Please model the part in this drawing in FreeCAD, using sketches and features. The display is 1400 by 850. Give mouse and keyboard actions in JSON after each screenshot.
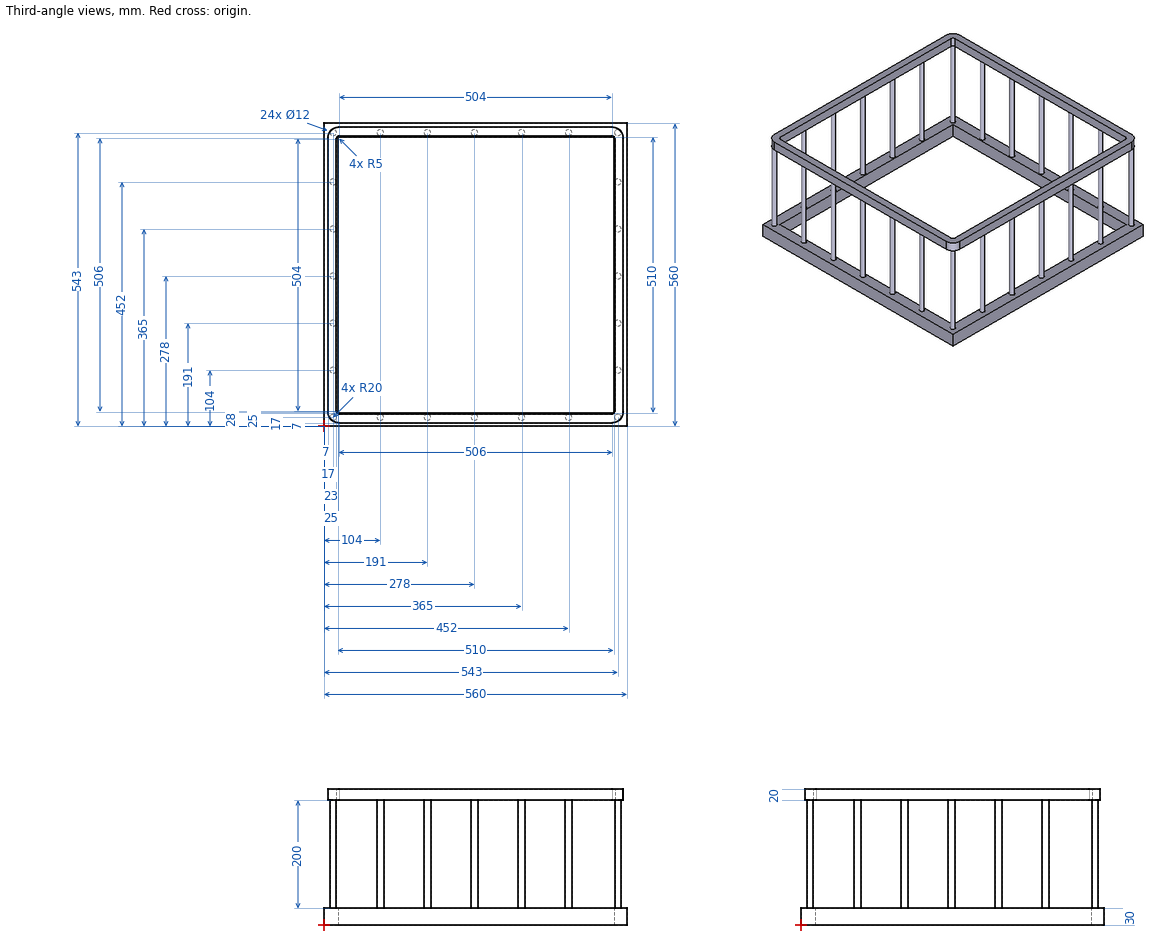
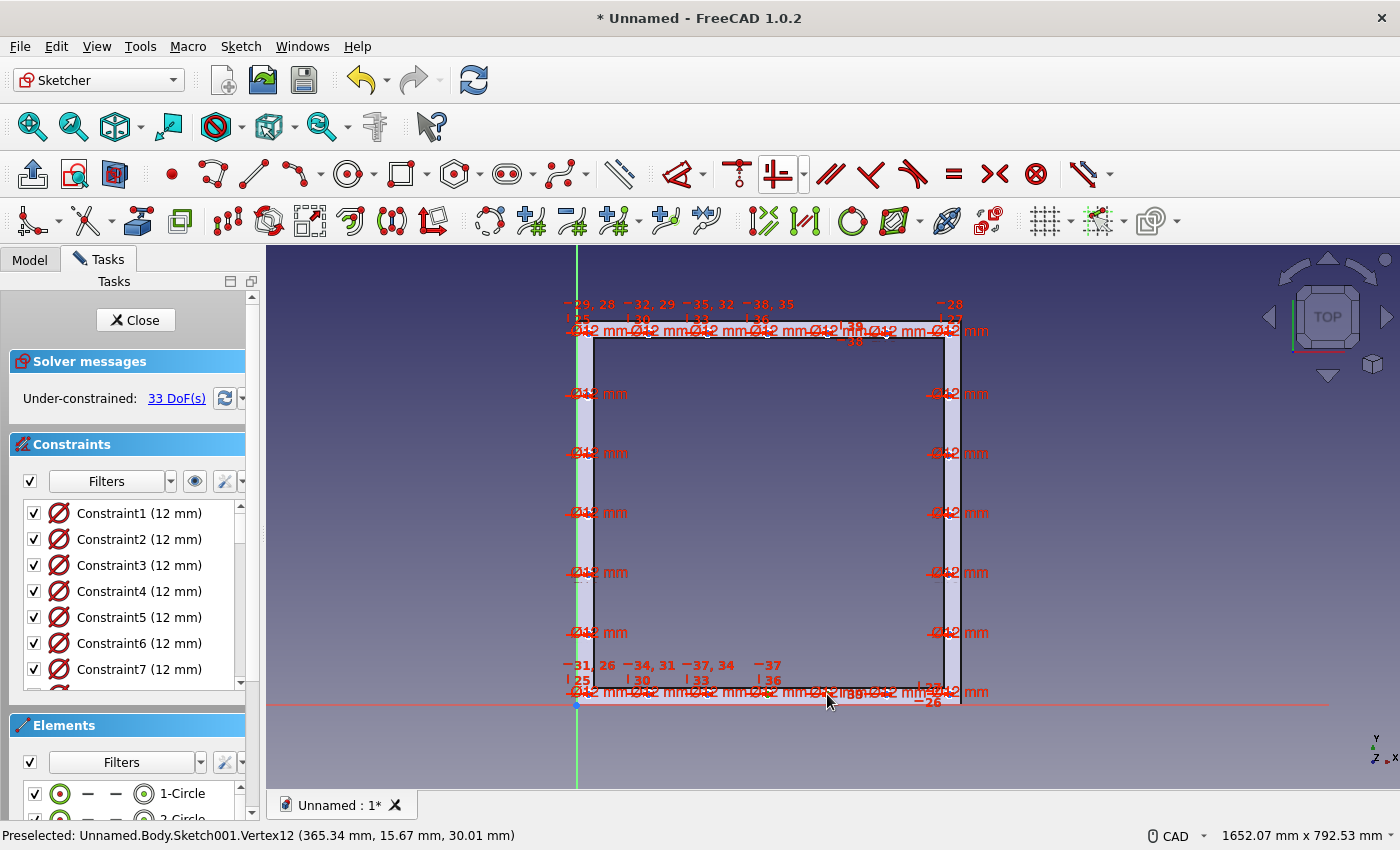
{"action": "key", "text": "h"}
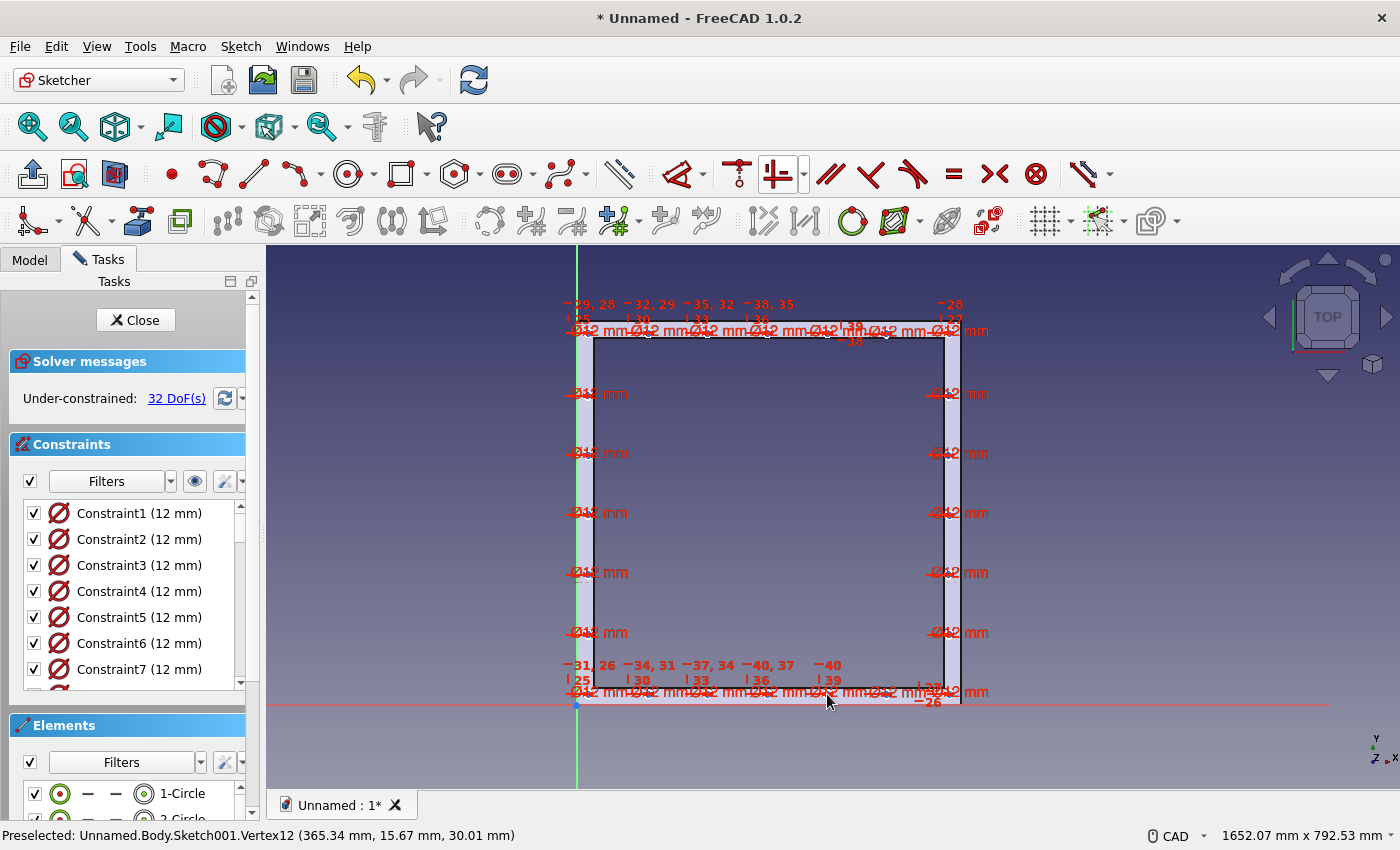
{"action": "left_click", "coordinate": [827, 333]}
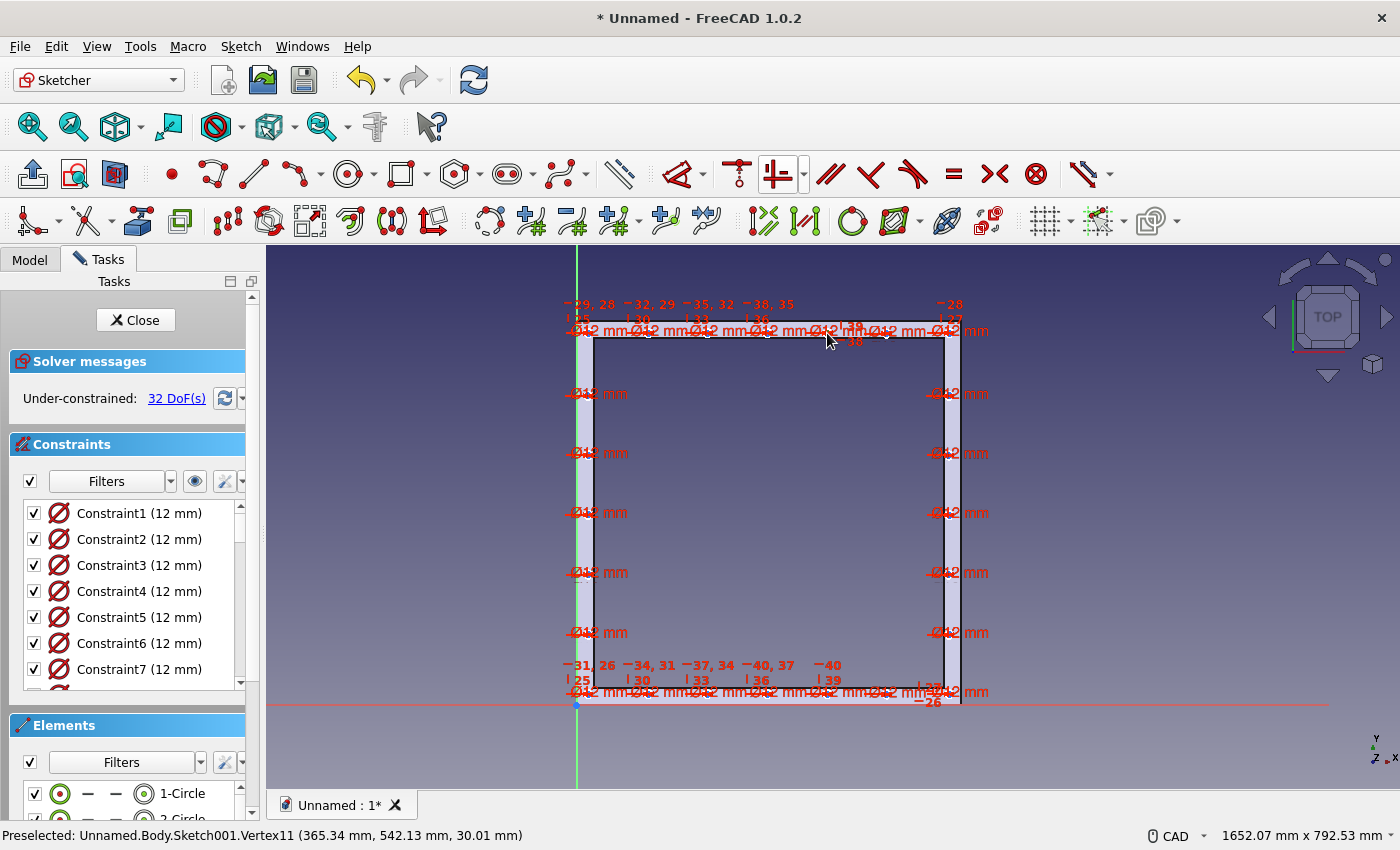
{"action": "left_click", "coordinate": [886, 334]}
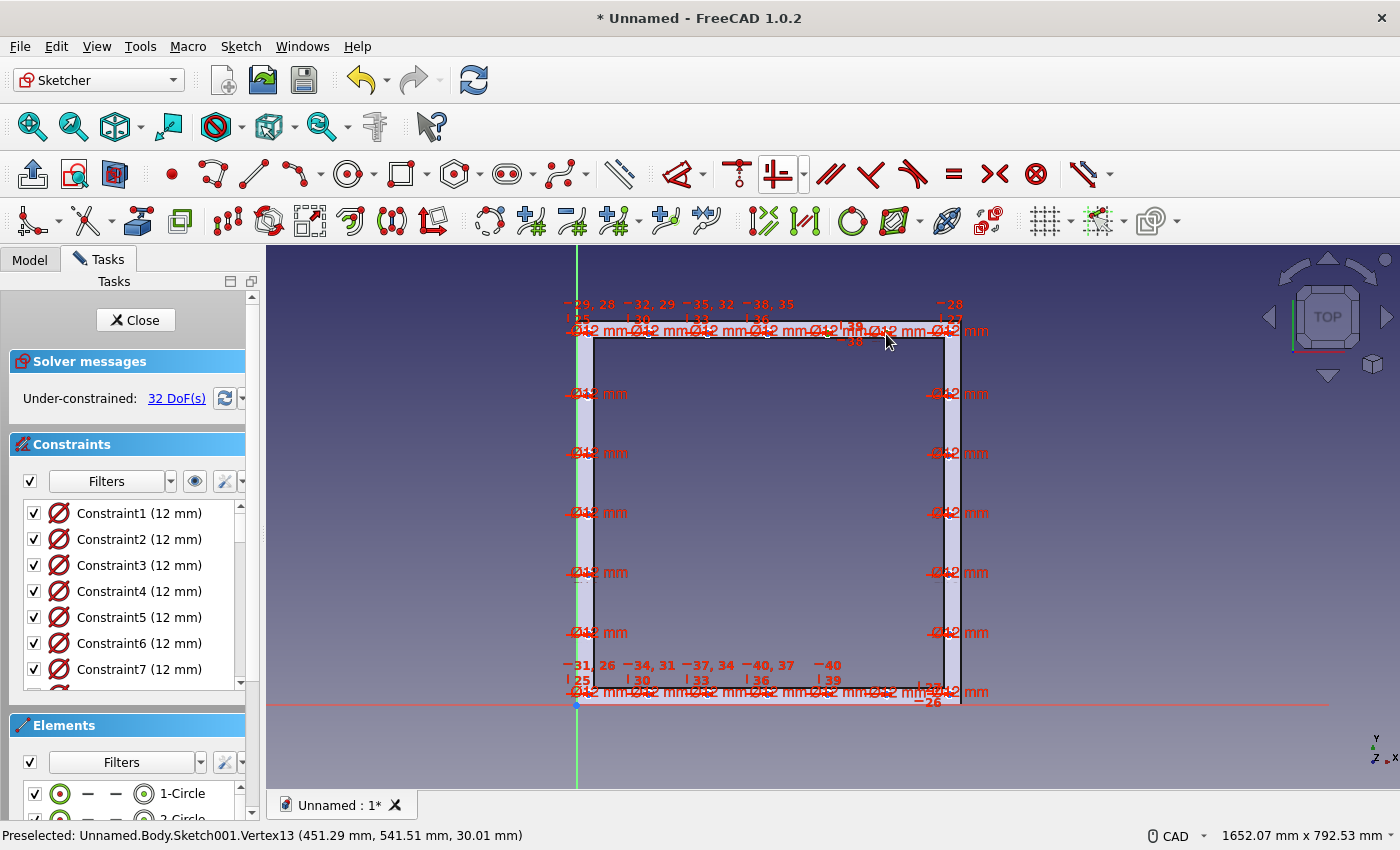
{"action": "left_click", "coordinate": [804, 174]}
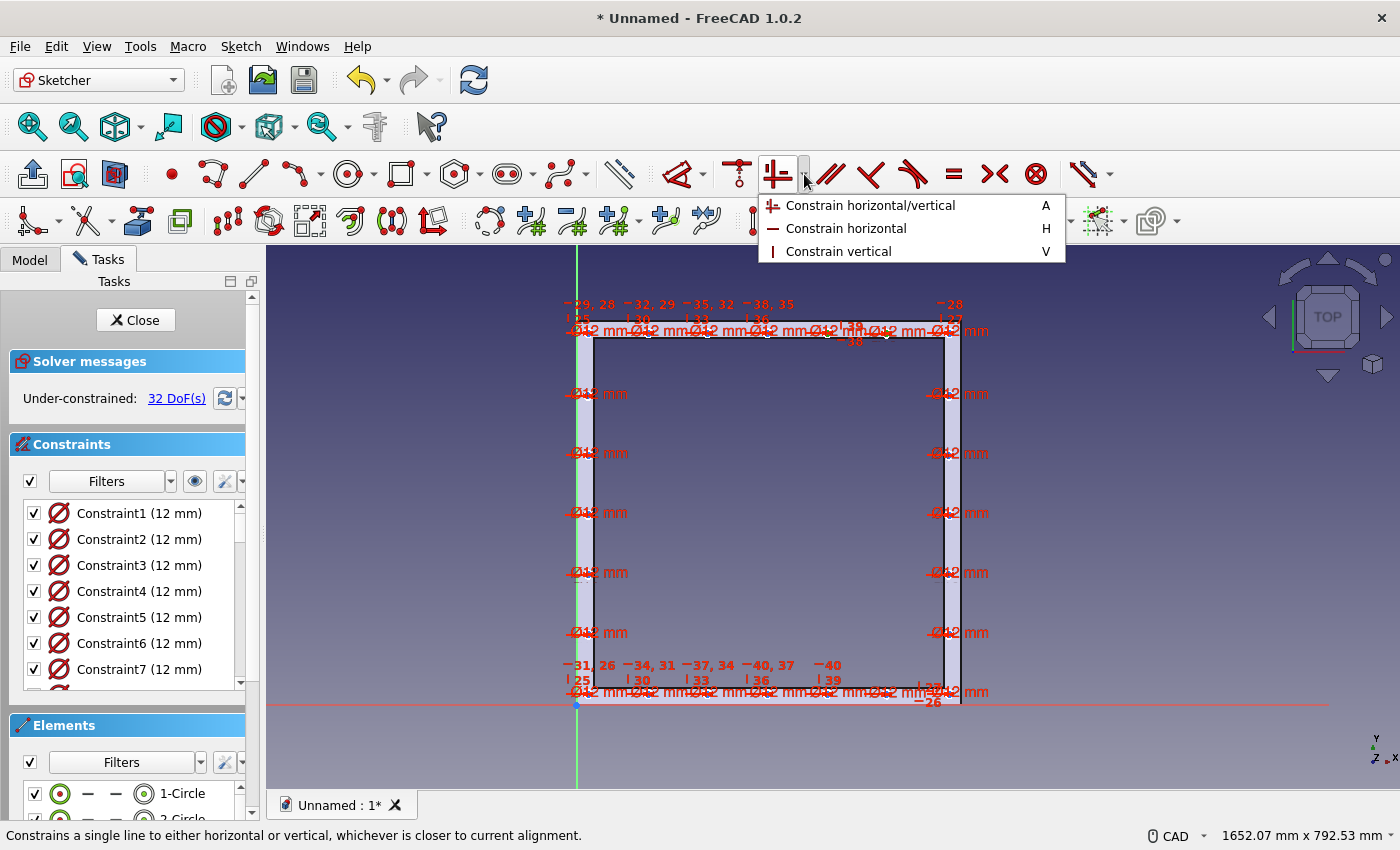
{"action": "left_click", "coordinate": [912, 228]}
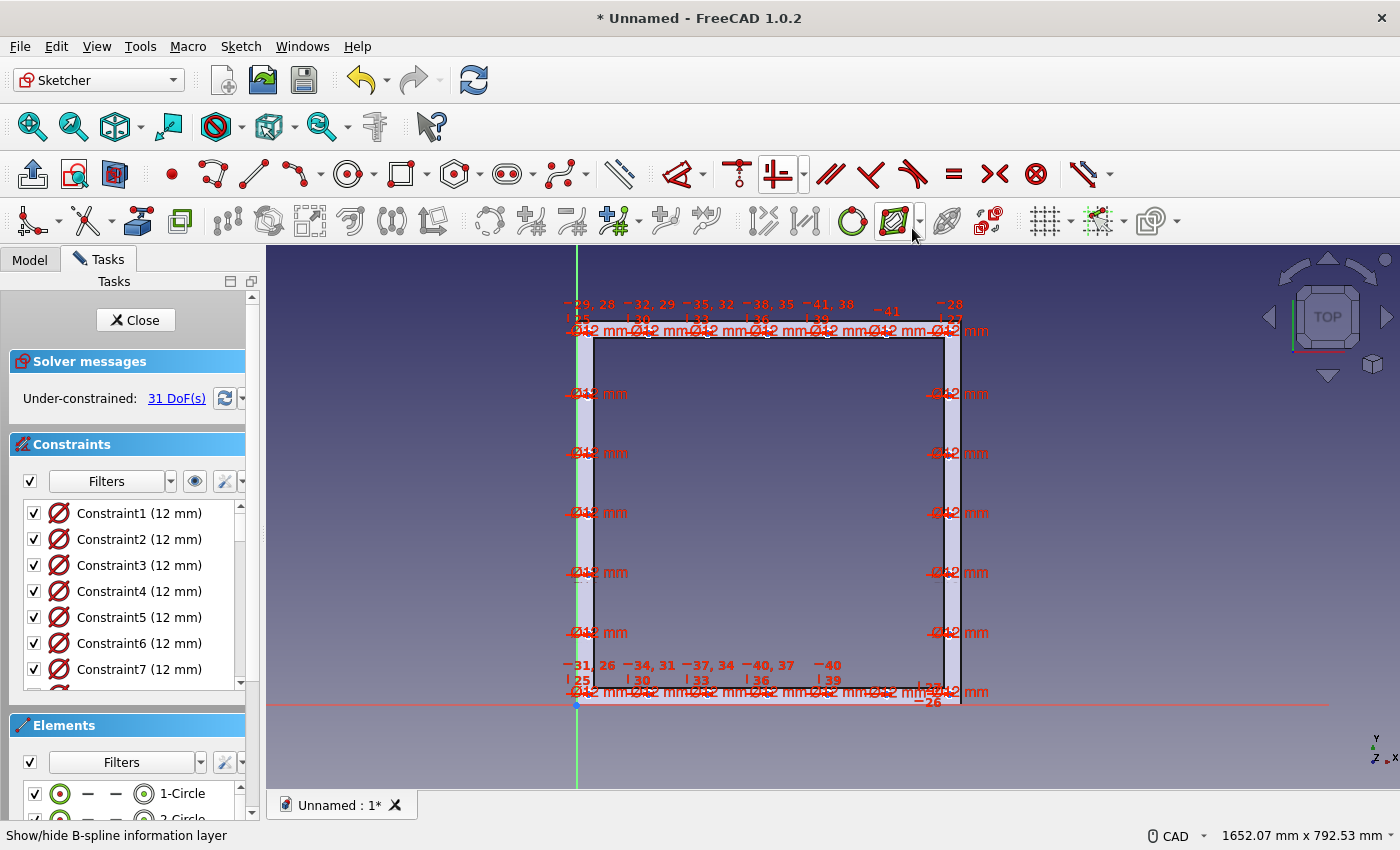
{"action": "left_click", "coordinate": [827, 694]}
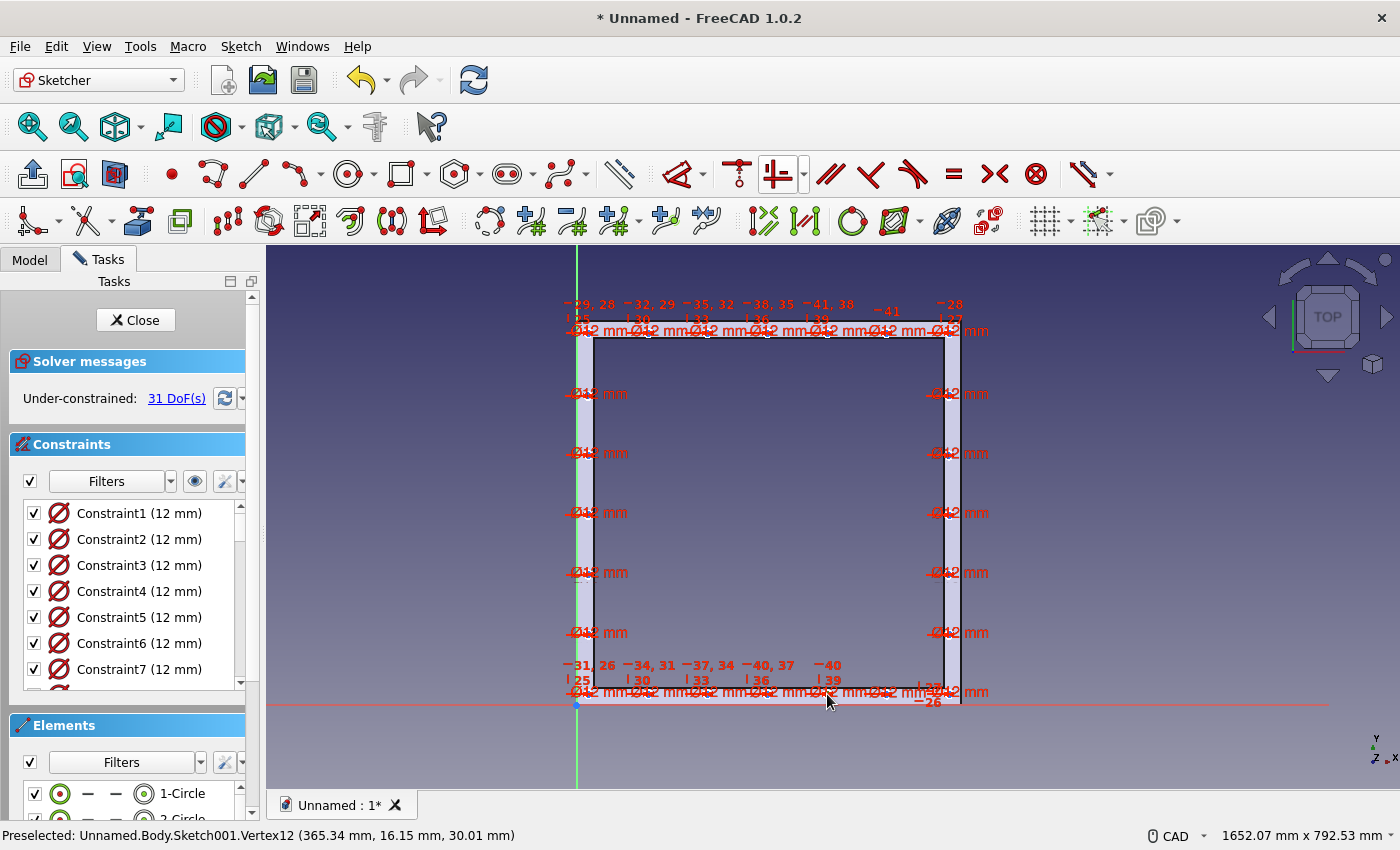
{"action": "left_click", "coordinate": [887, 694]}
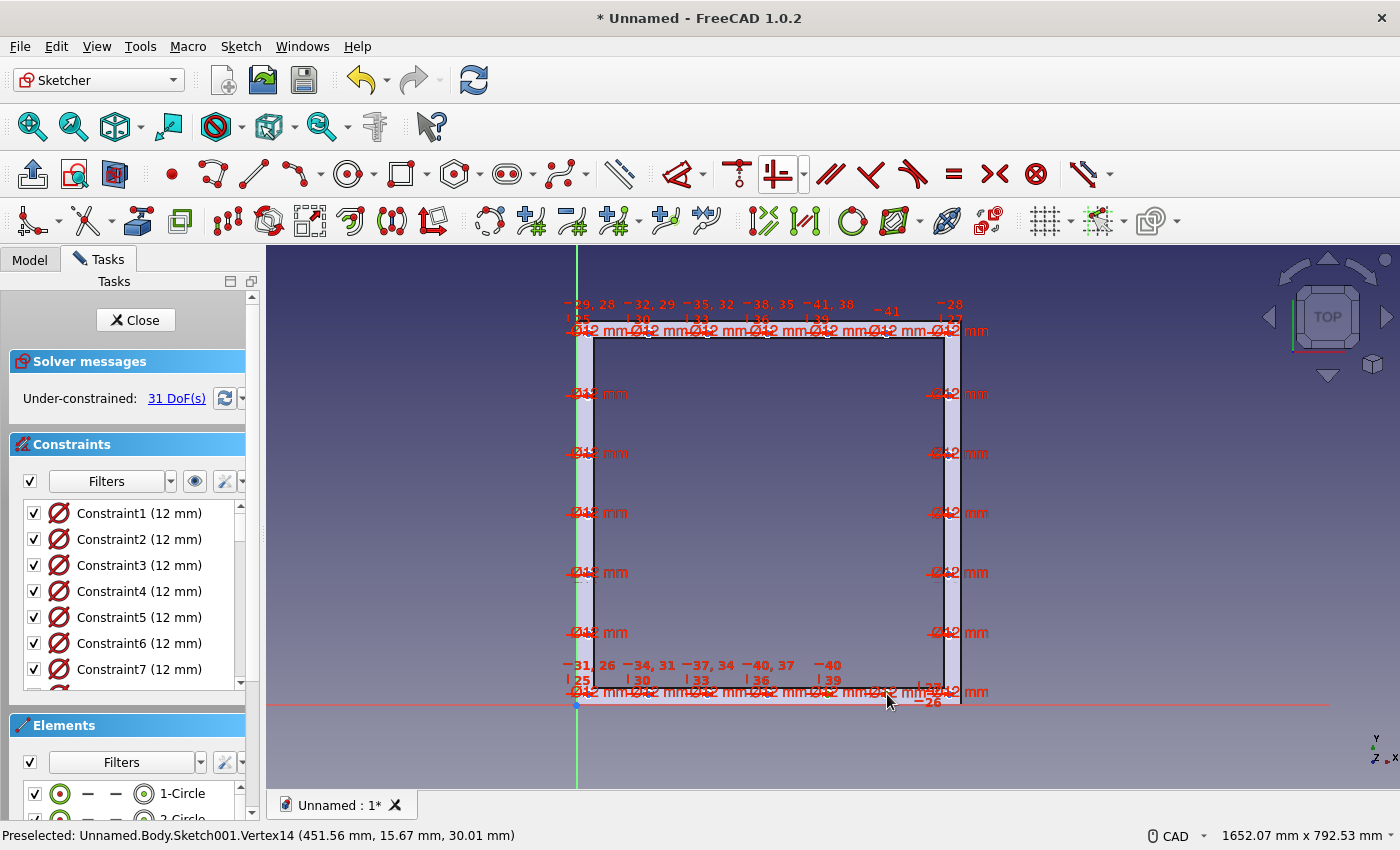
{"action": "key", "text": "h"}